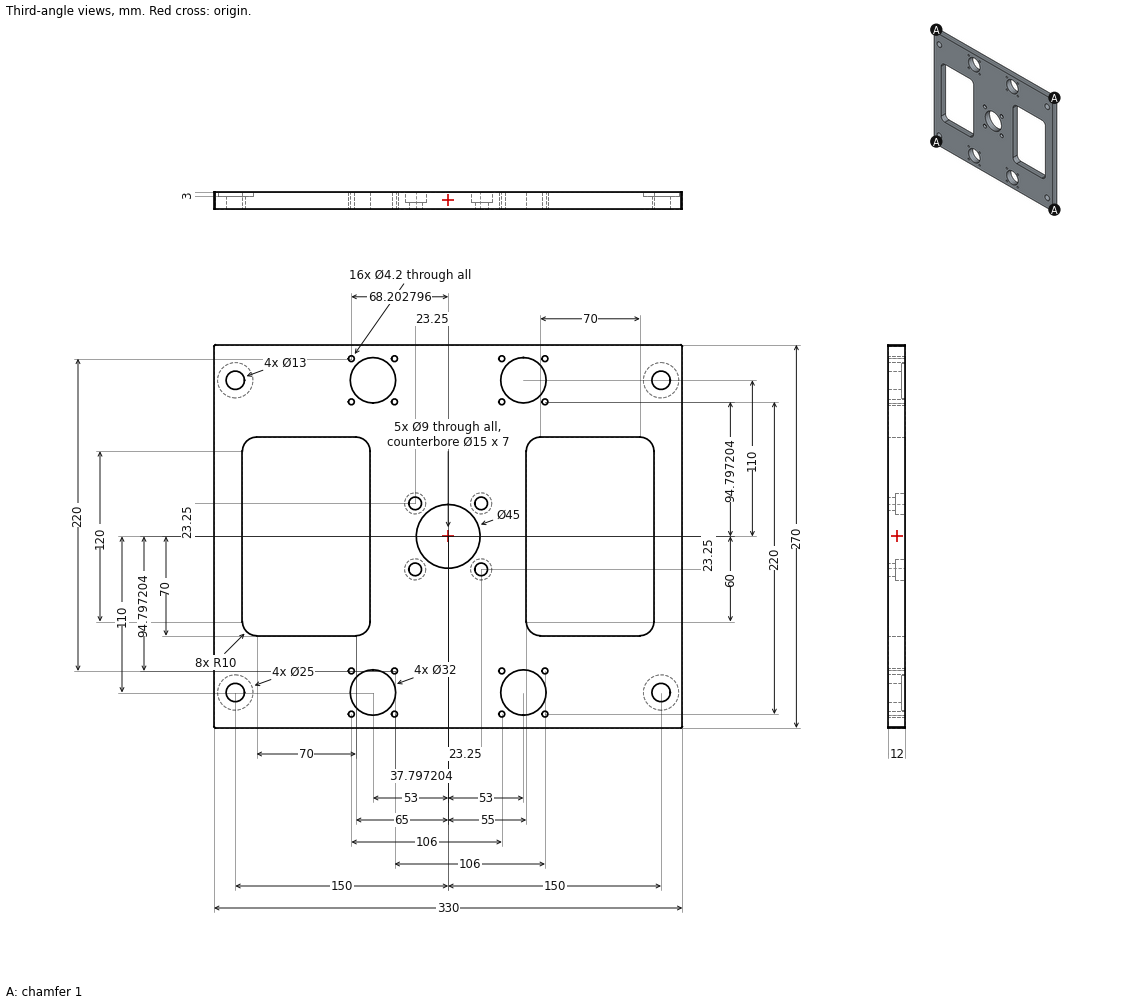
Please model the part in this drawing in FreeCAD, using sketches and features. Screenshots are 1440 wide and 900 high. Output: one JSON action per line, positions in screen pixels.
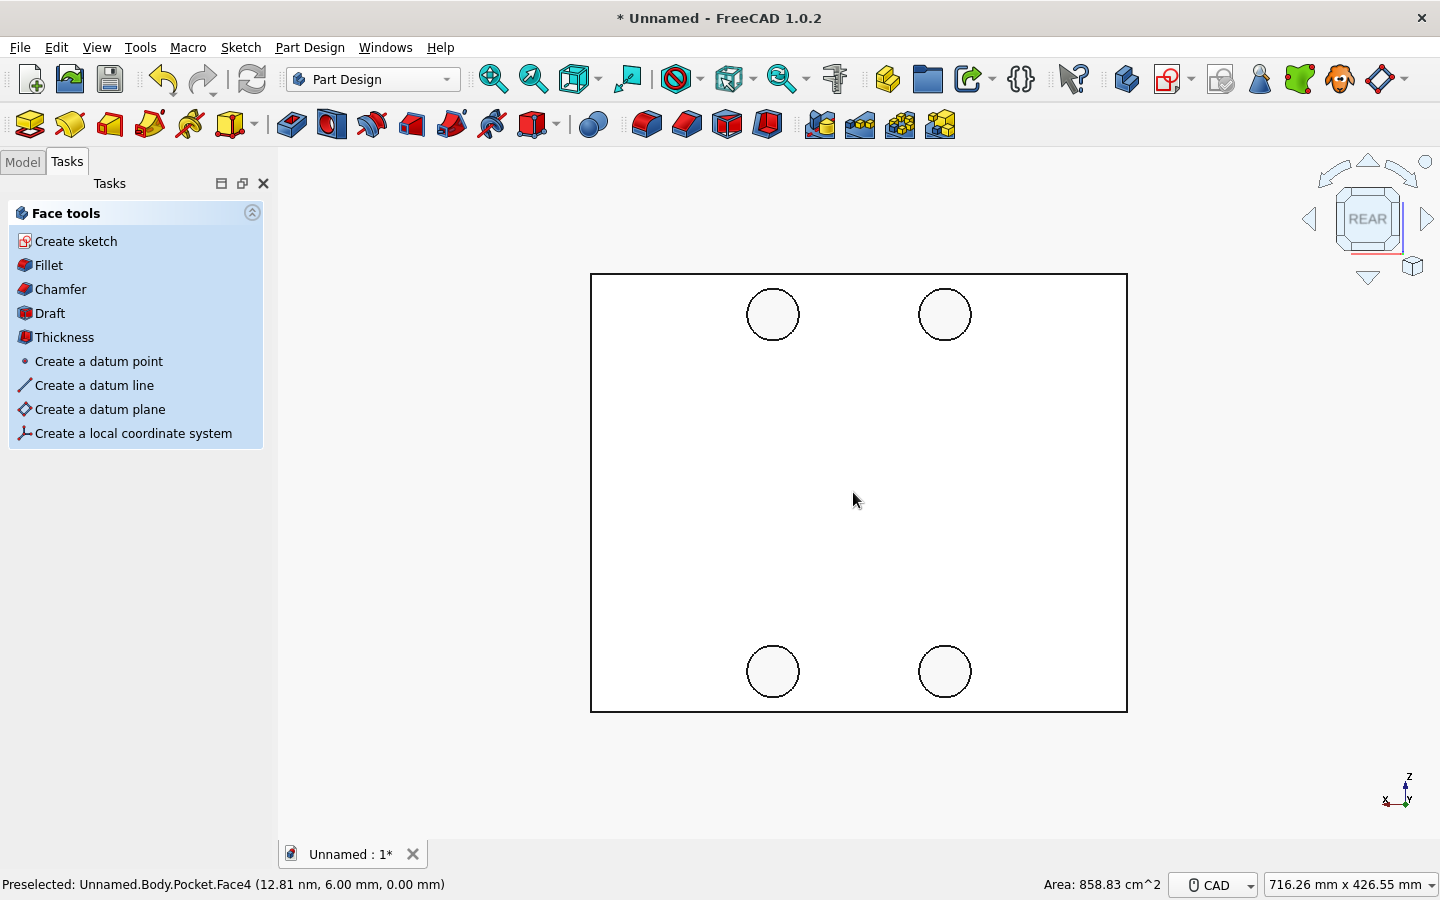
{"action": "left_click", "coordinate": [1168, 80]}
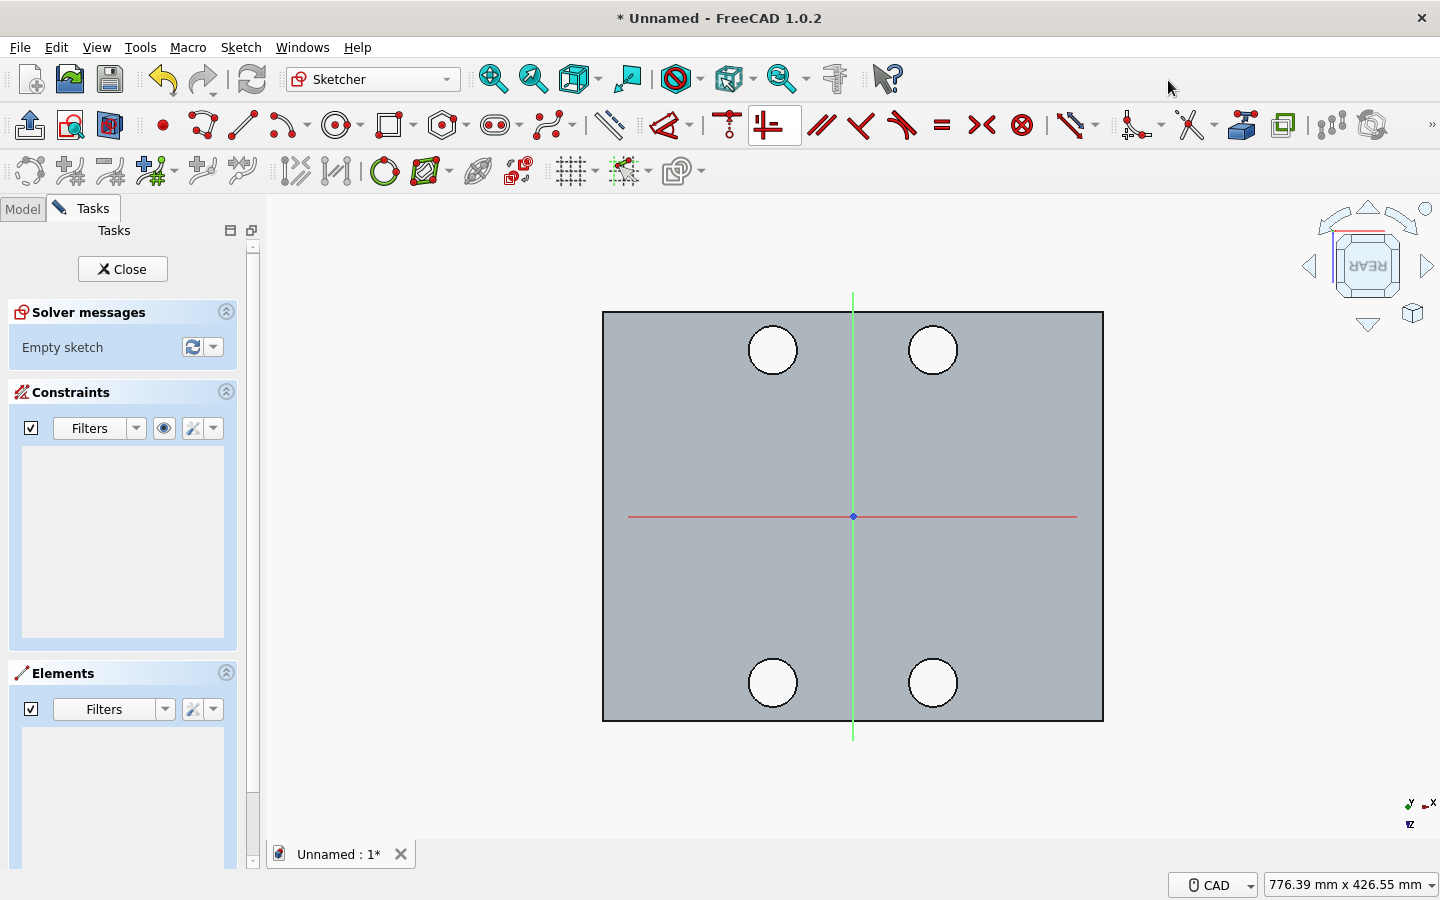
{"action": "scroll", "coordinate": [867, 516], "scroll_direction": "up", "scroll_amount": 9}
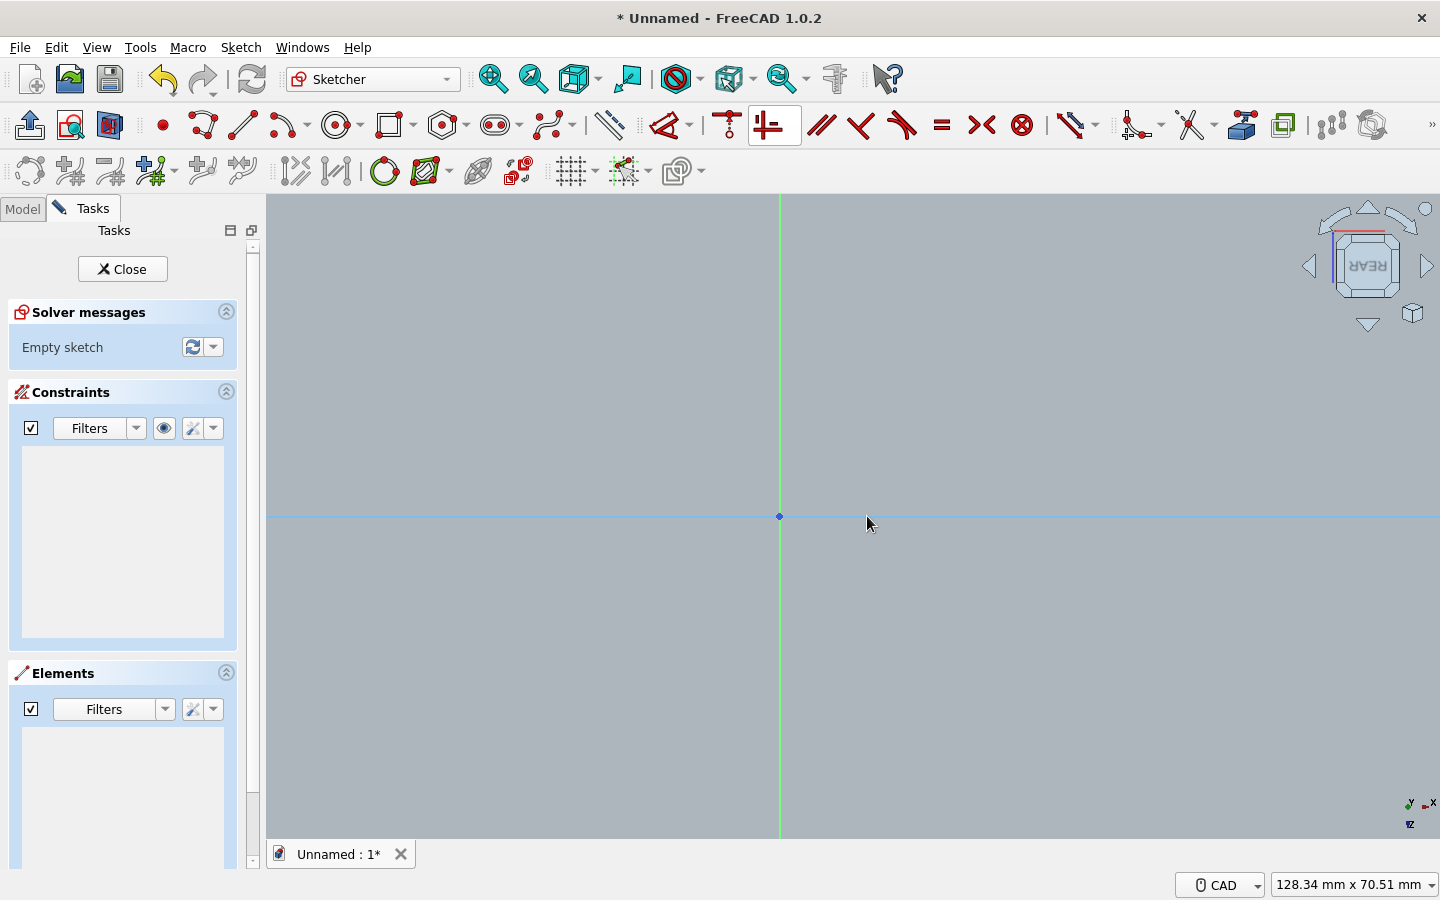
{"action": "left_click", "coordinate": [336, 126]}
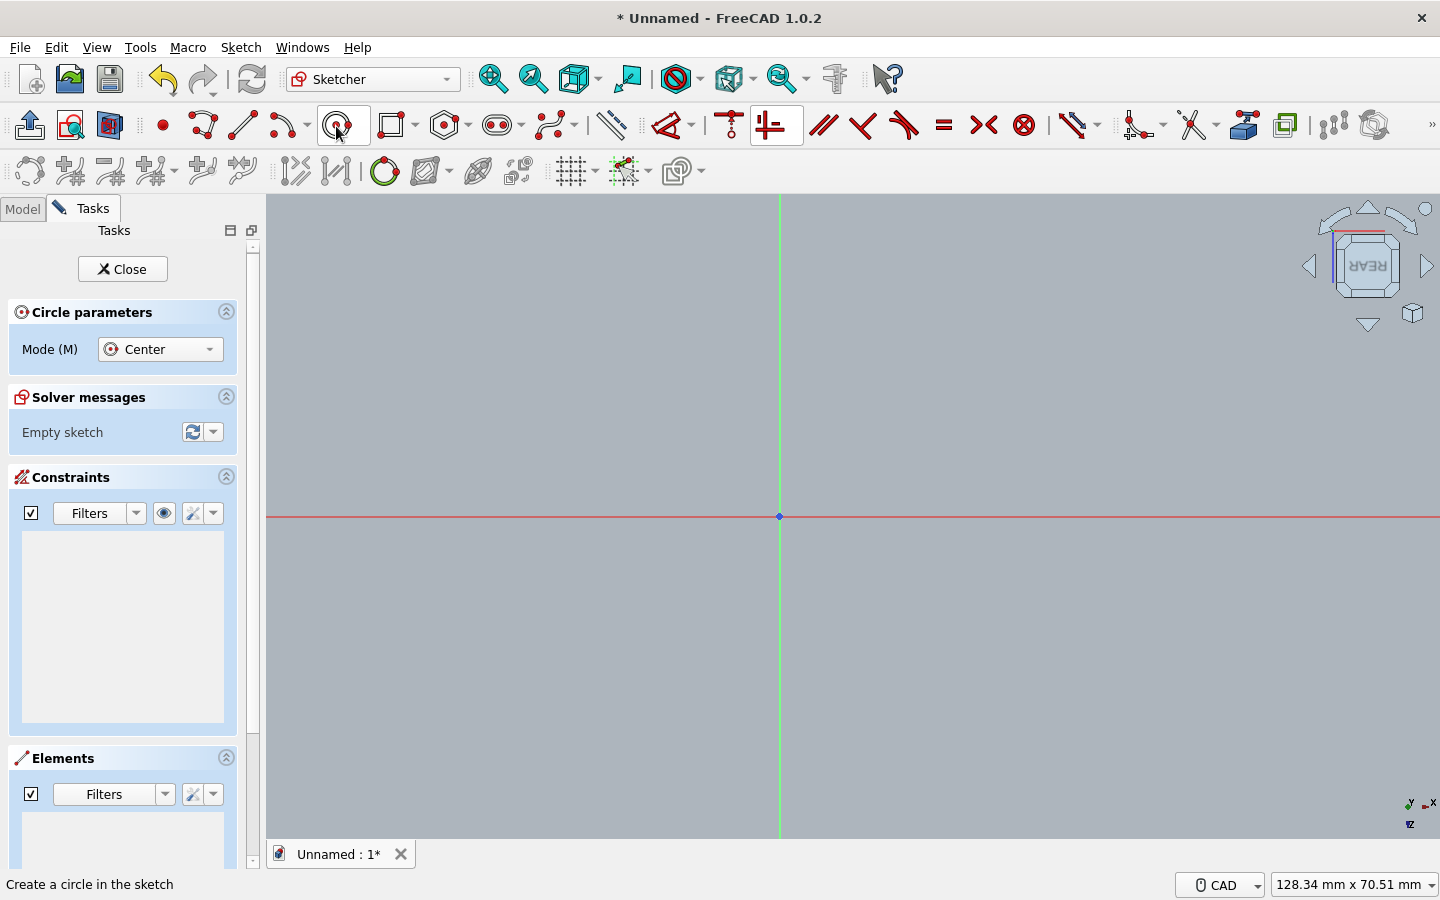
{"action": "left_click", "coordinate": [780, 516]}
{"action": "mouse_move", "coordinate": [925, 371]}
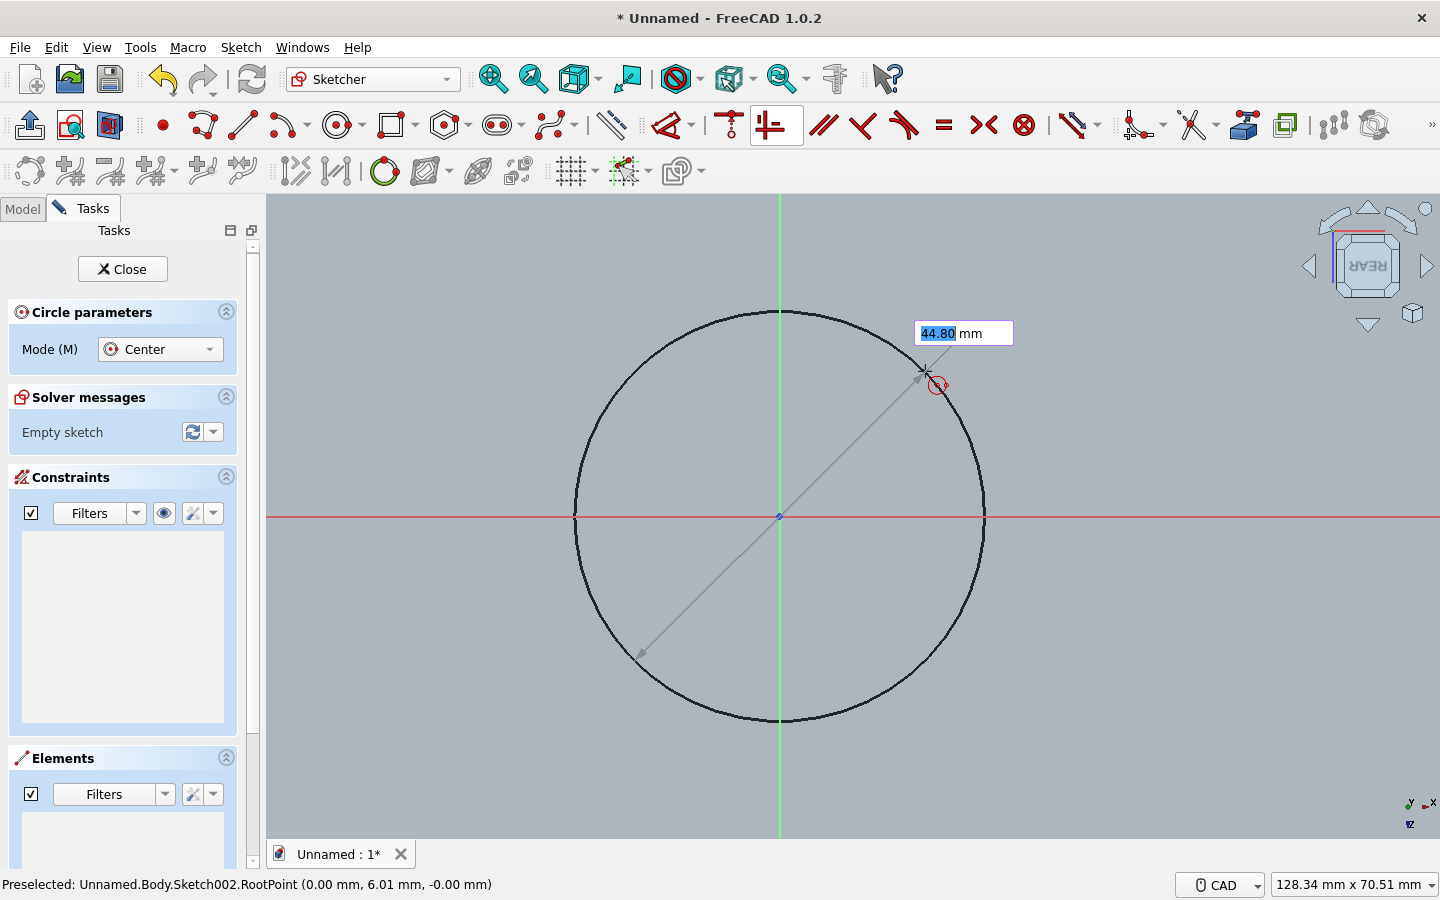
{"action": "type", "text": "45"}
{"action": "key", "text": "Return"}
{"action": "key", "text": "Escape"}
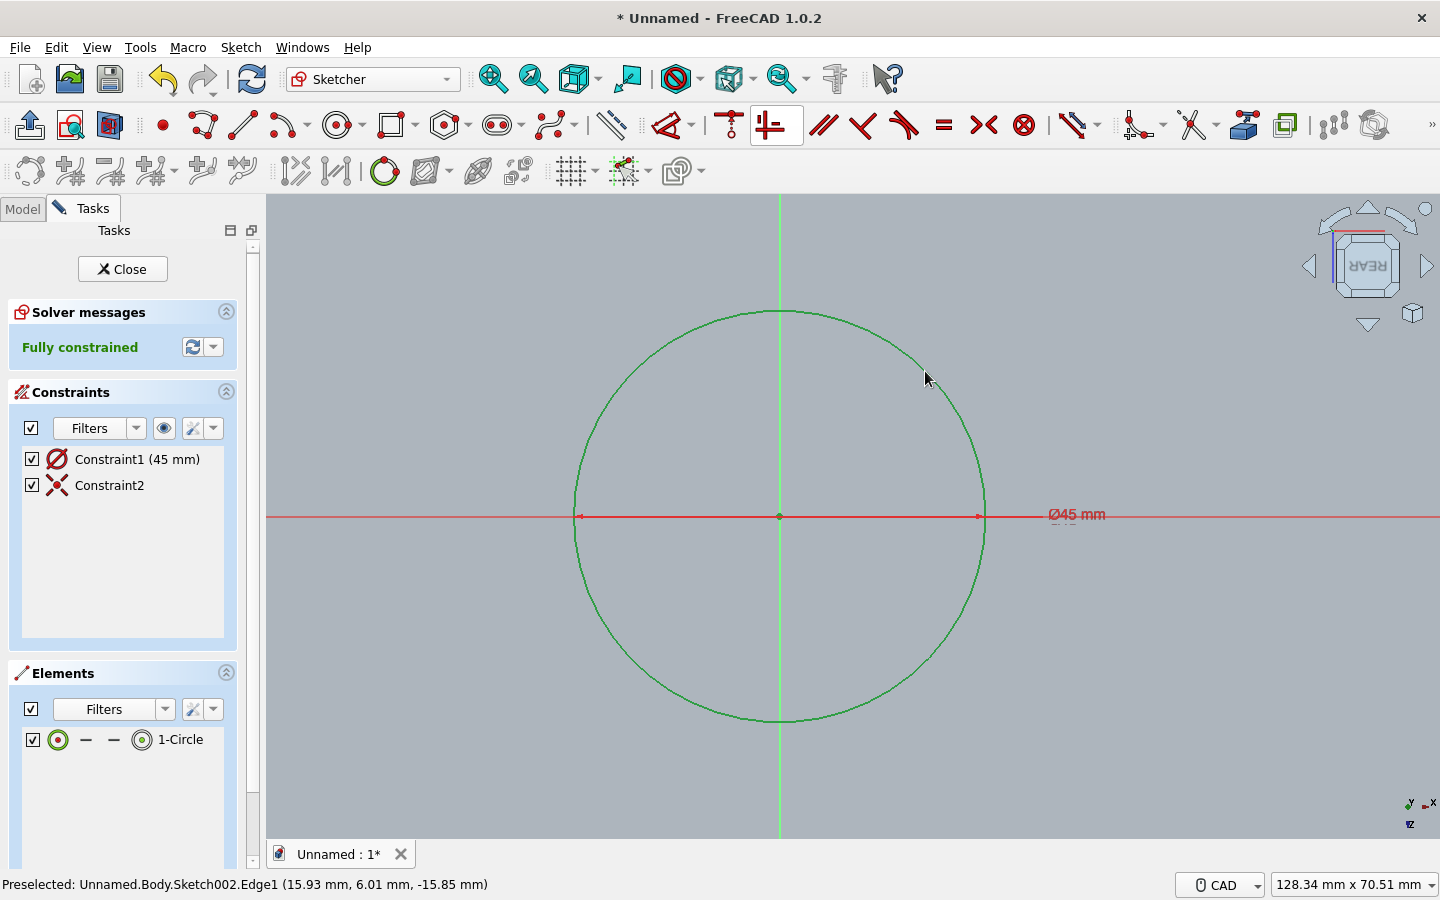
{"action": "left_click", "coordinate": [123, 269]}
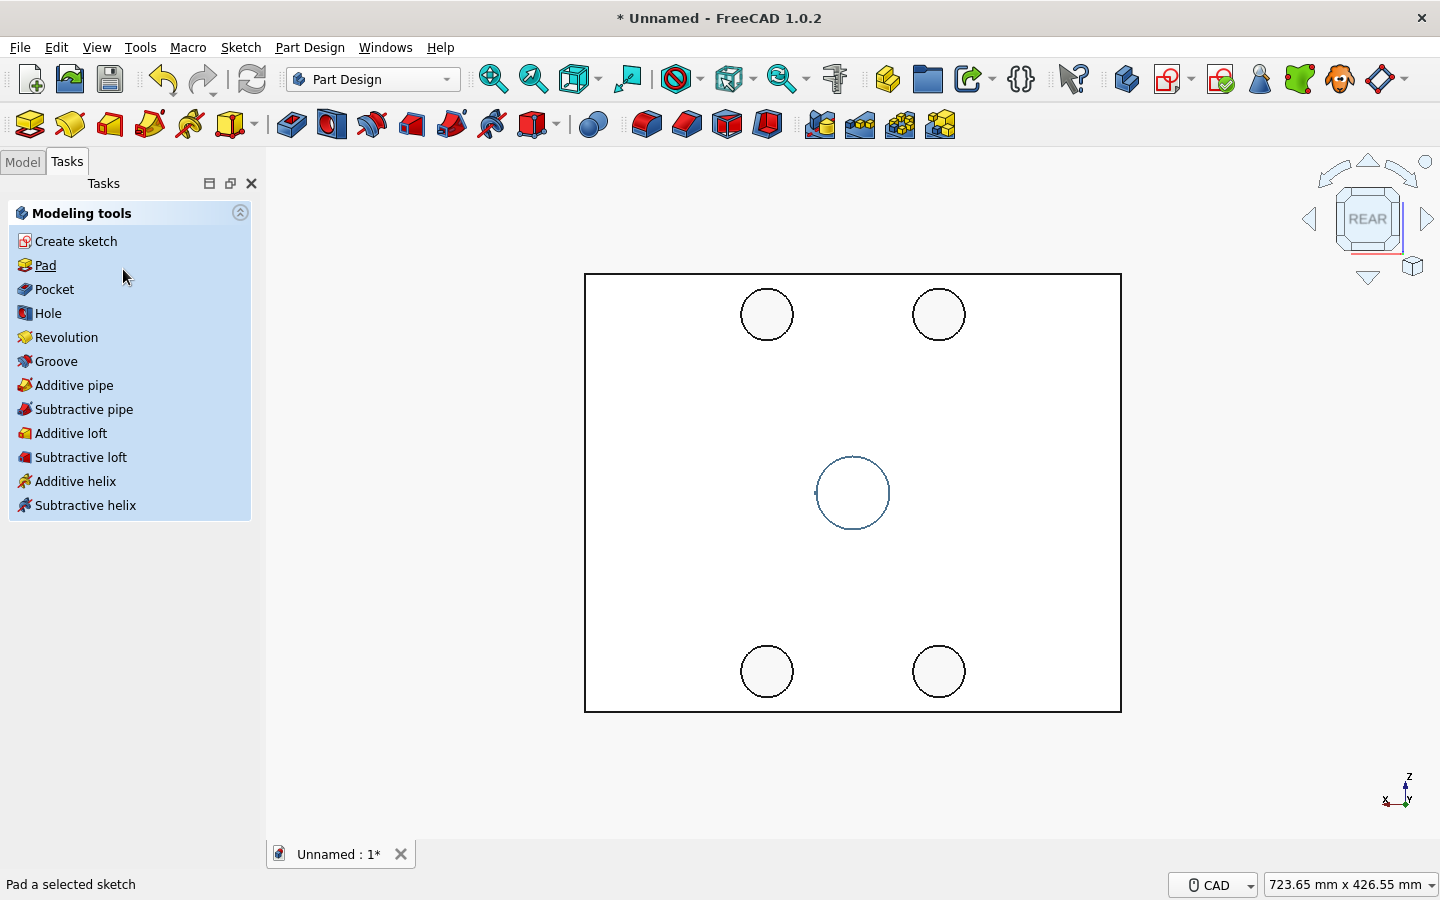
{"action": "left_click", "coordinate": [292, 124]}